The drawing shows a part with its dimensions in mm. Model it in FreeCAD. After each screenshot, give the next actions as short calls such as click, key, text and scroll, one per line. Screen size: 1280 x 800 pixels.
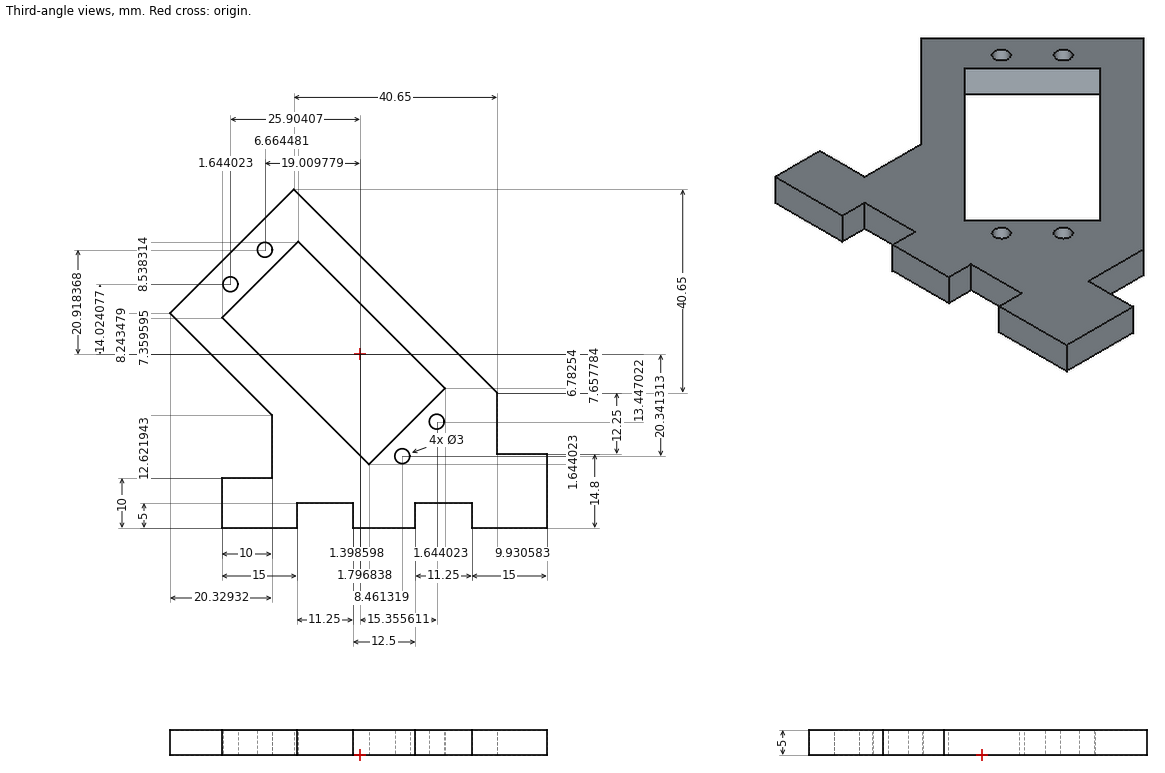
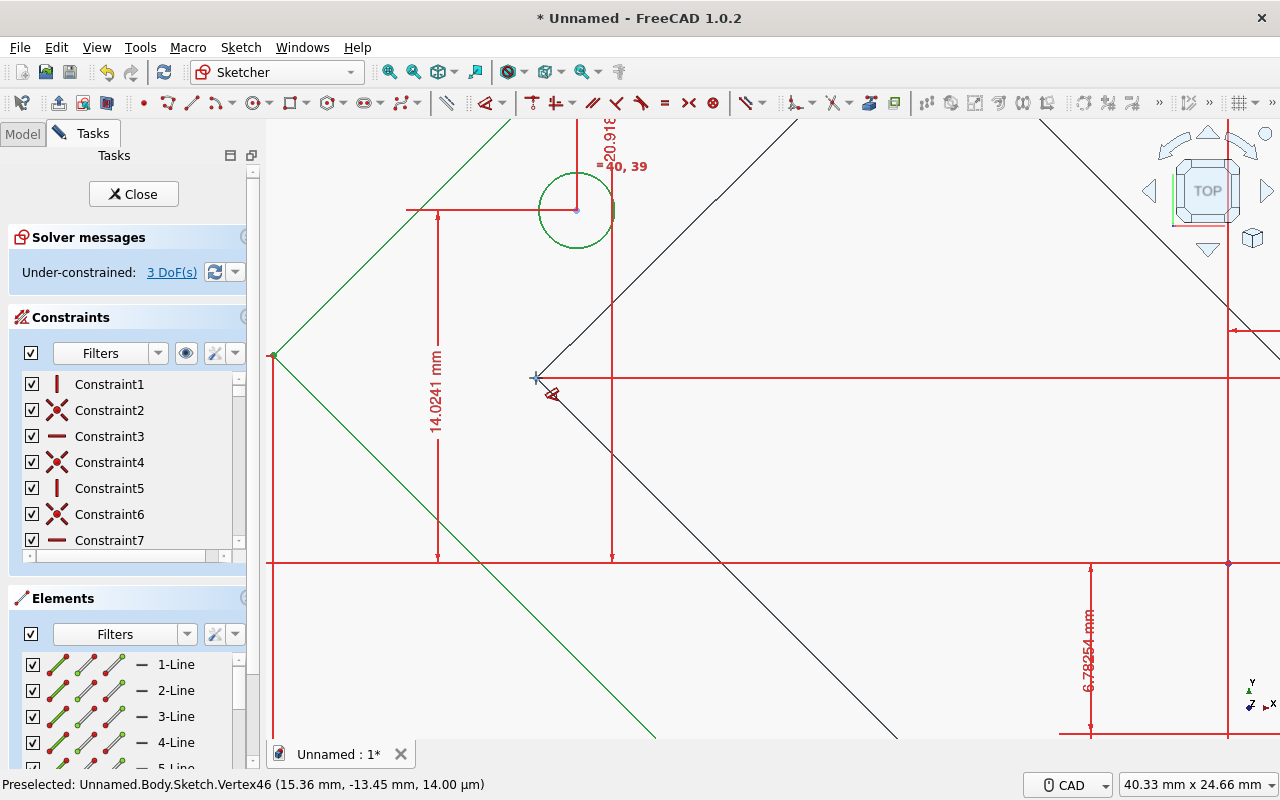
click(537, 378)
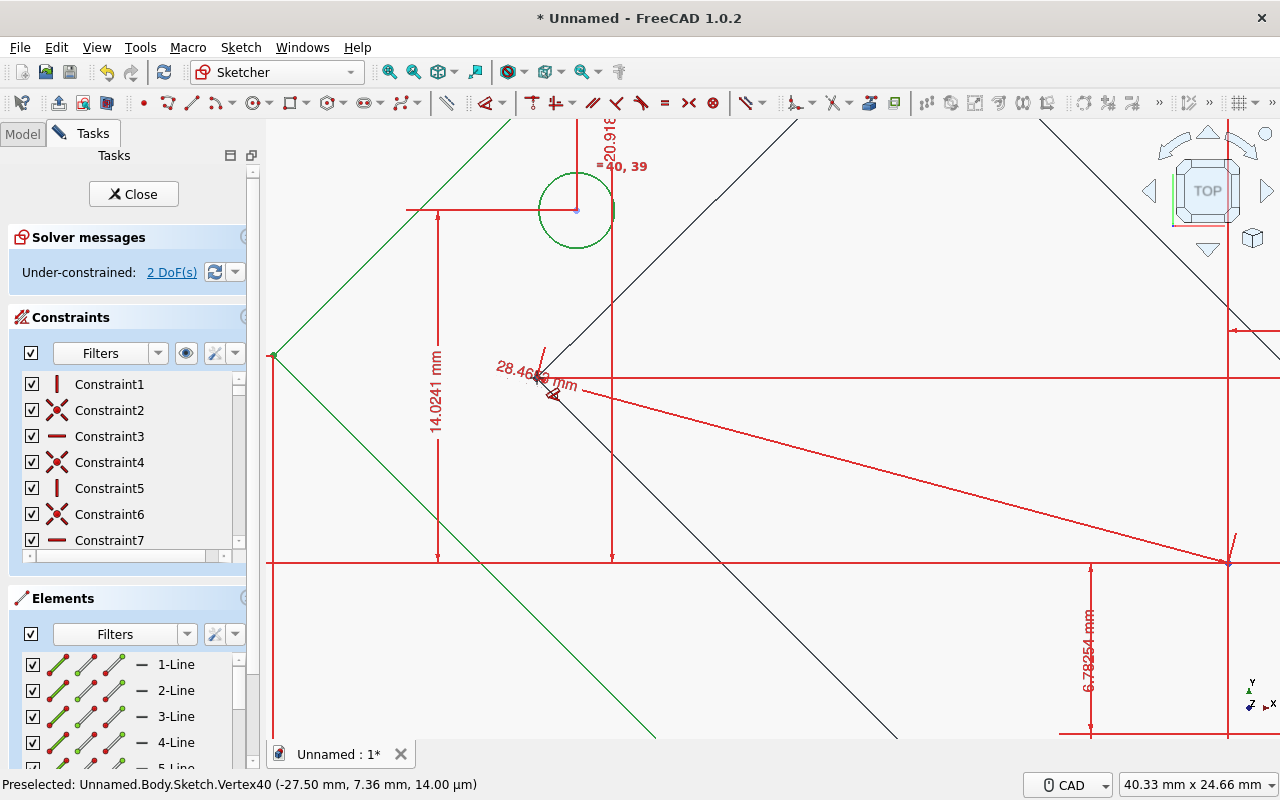
click(577, 210)
click(548, 412)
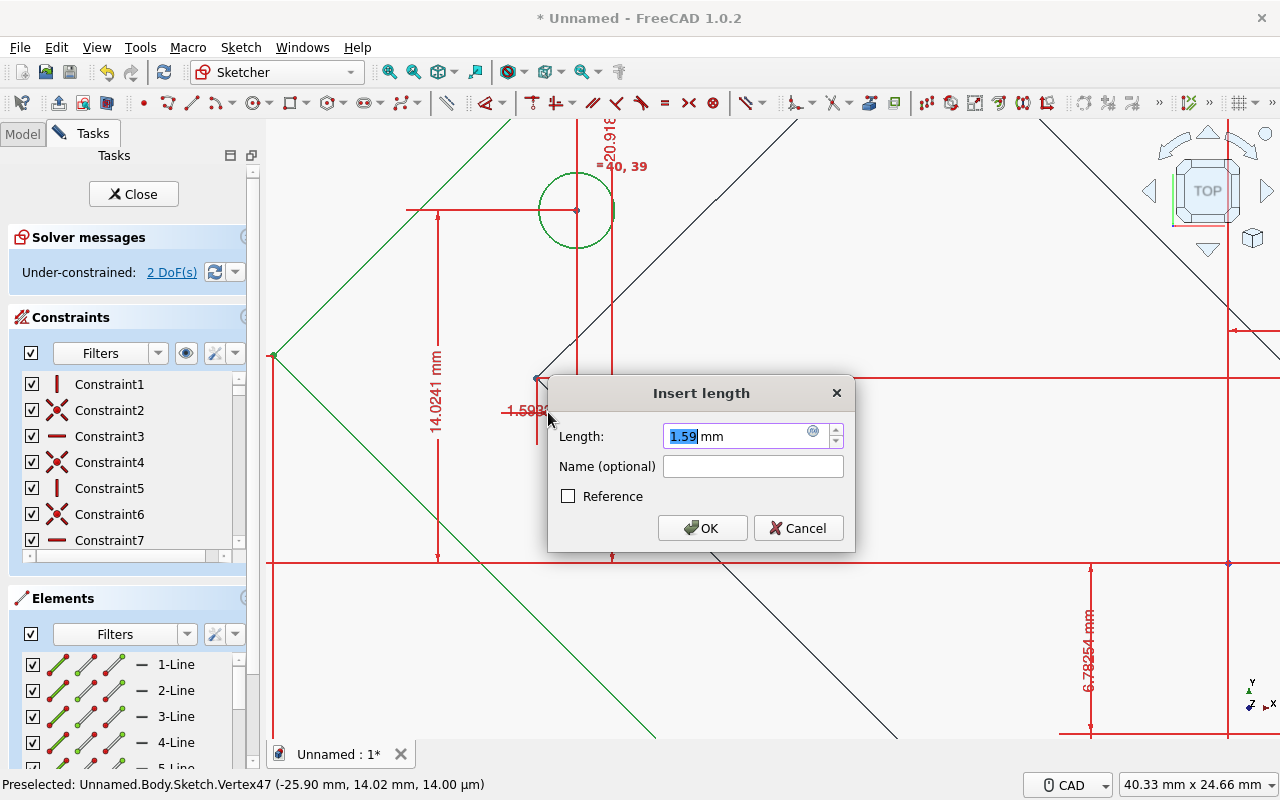
text(1.644023)
key(Return)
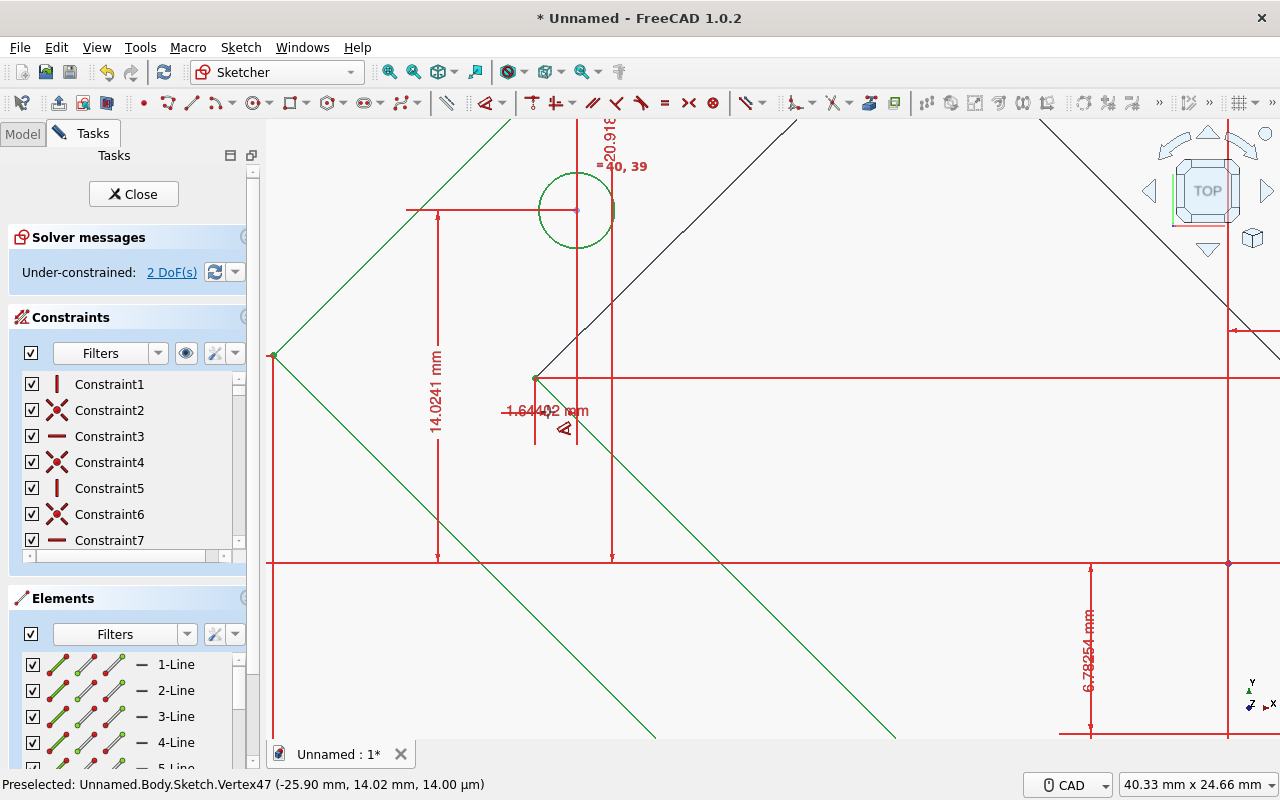
scroll(536, 378, down, 7)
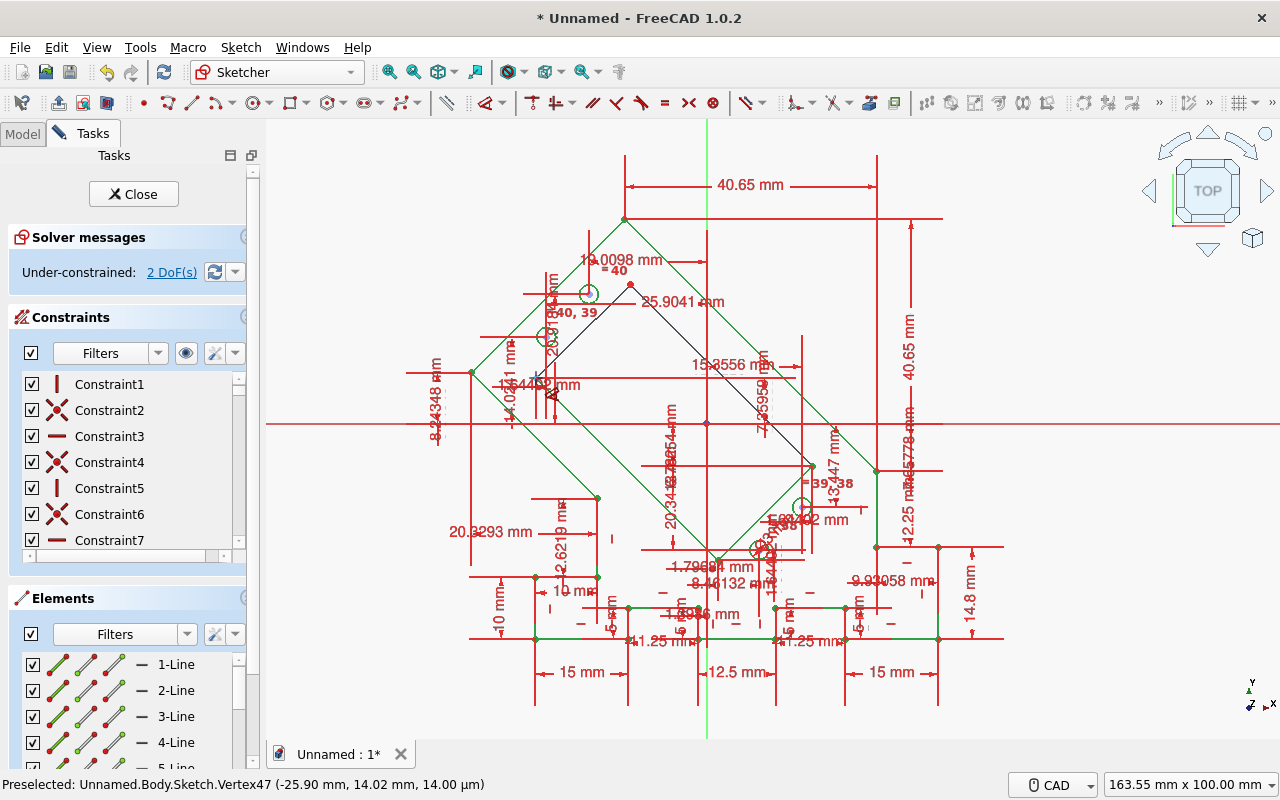
click(631, 285)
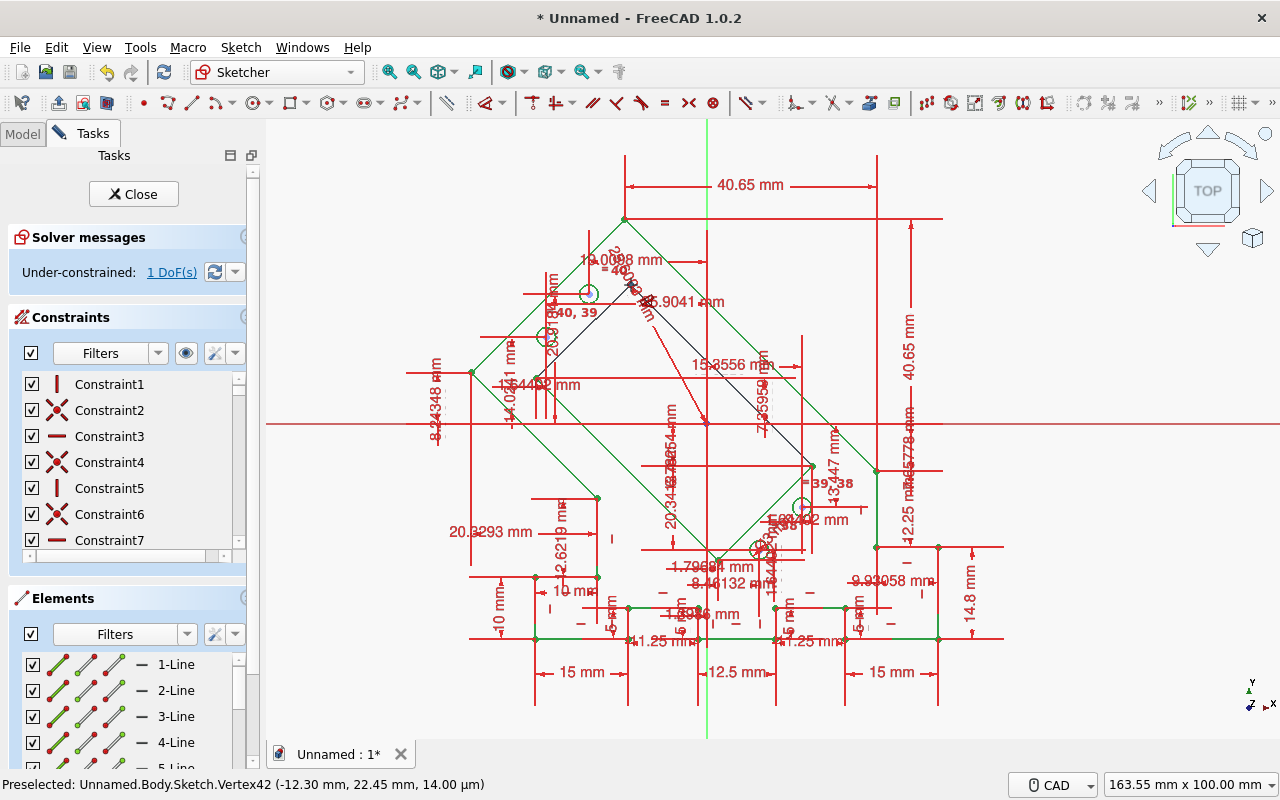
click(546, 337)
click(512, 293)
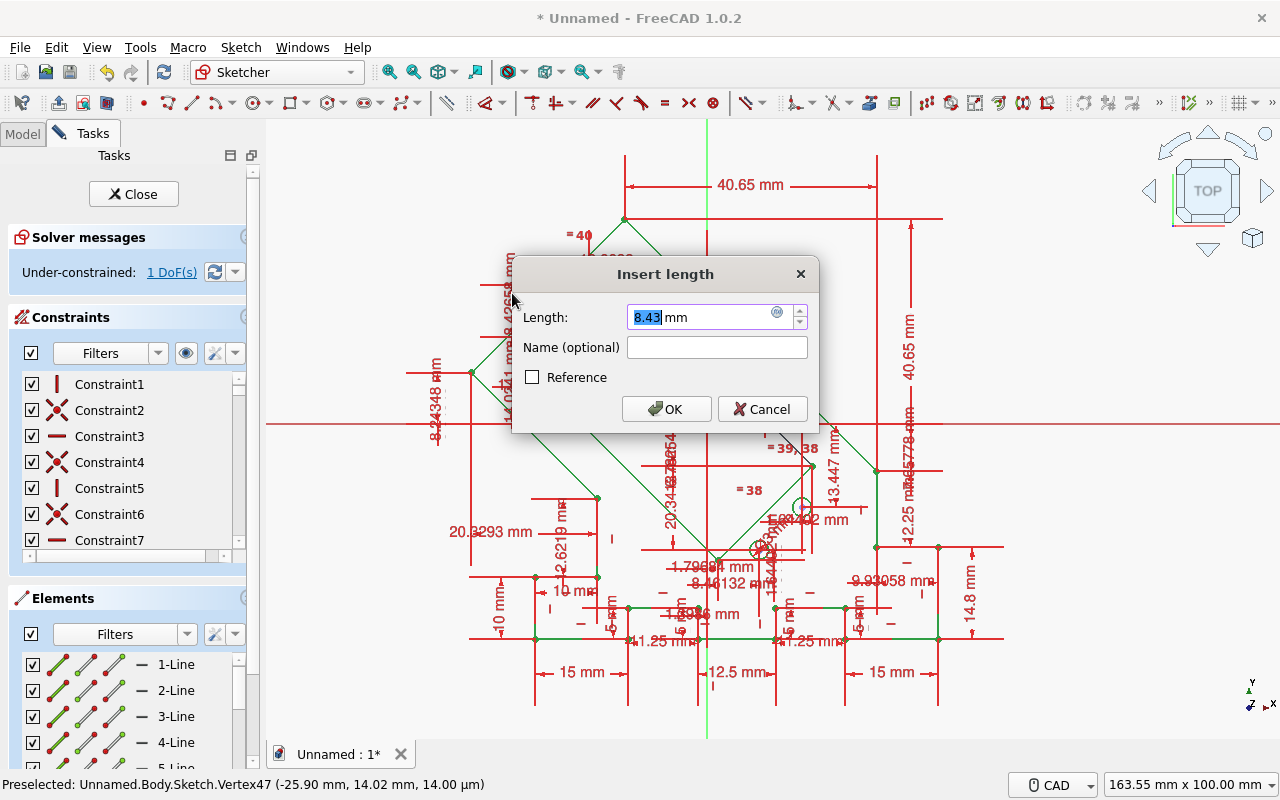
text(8.538314)
key(Return)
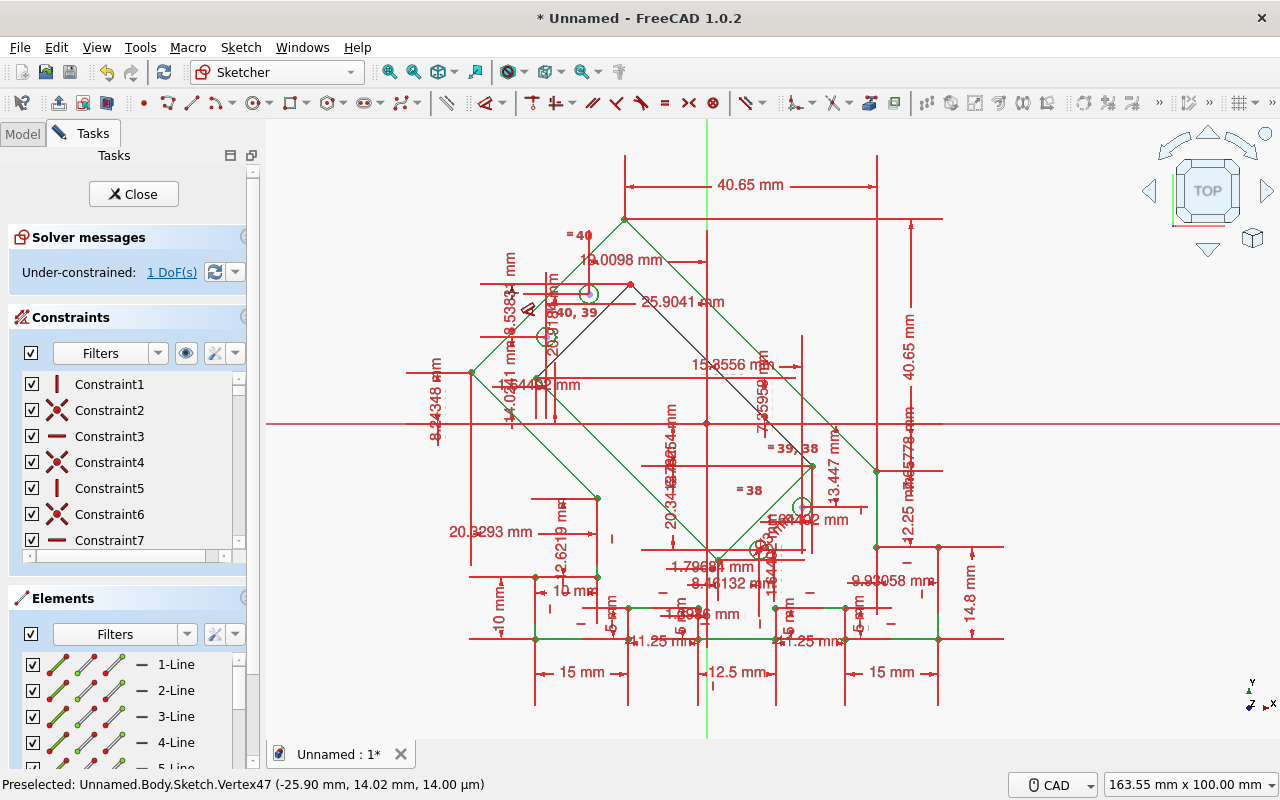
click(631, 284)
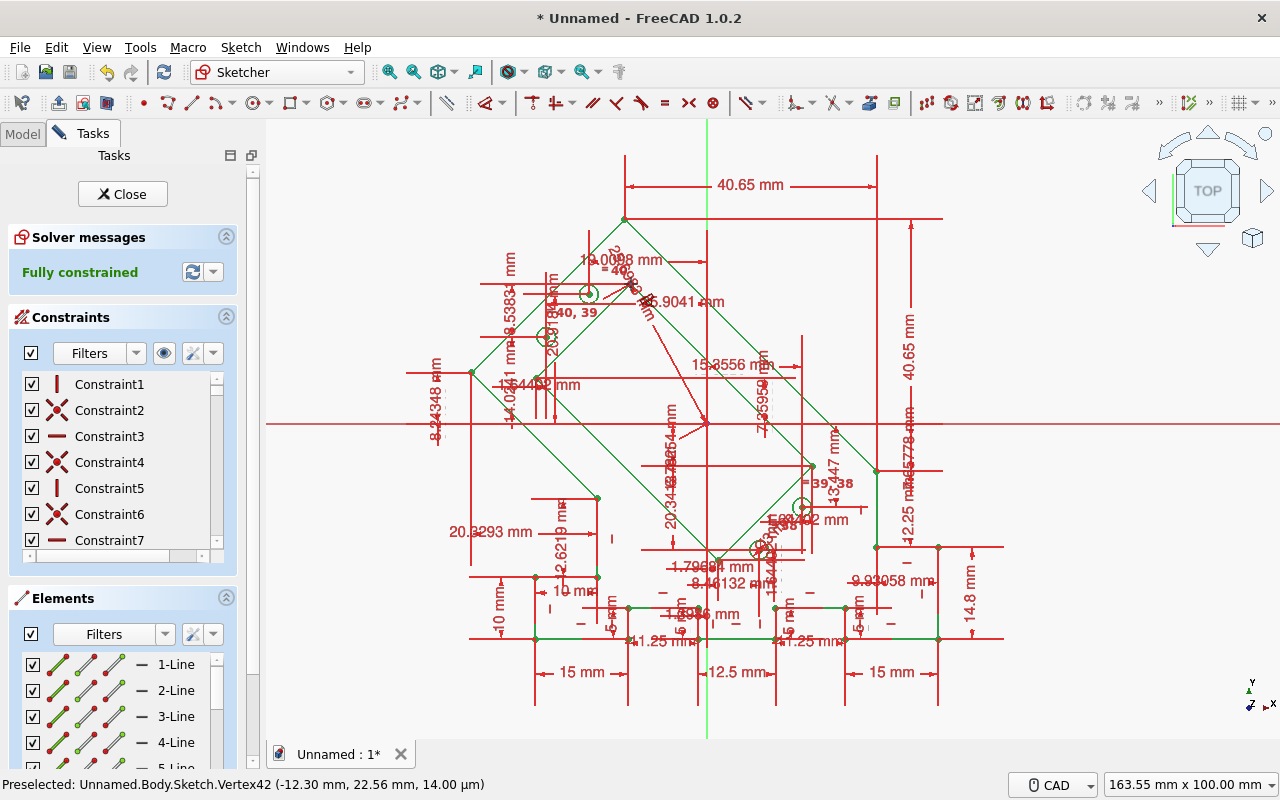
click(589, 294)
click(595, 226)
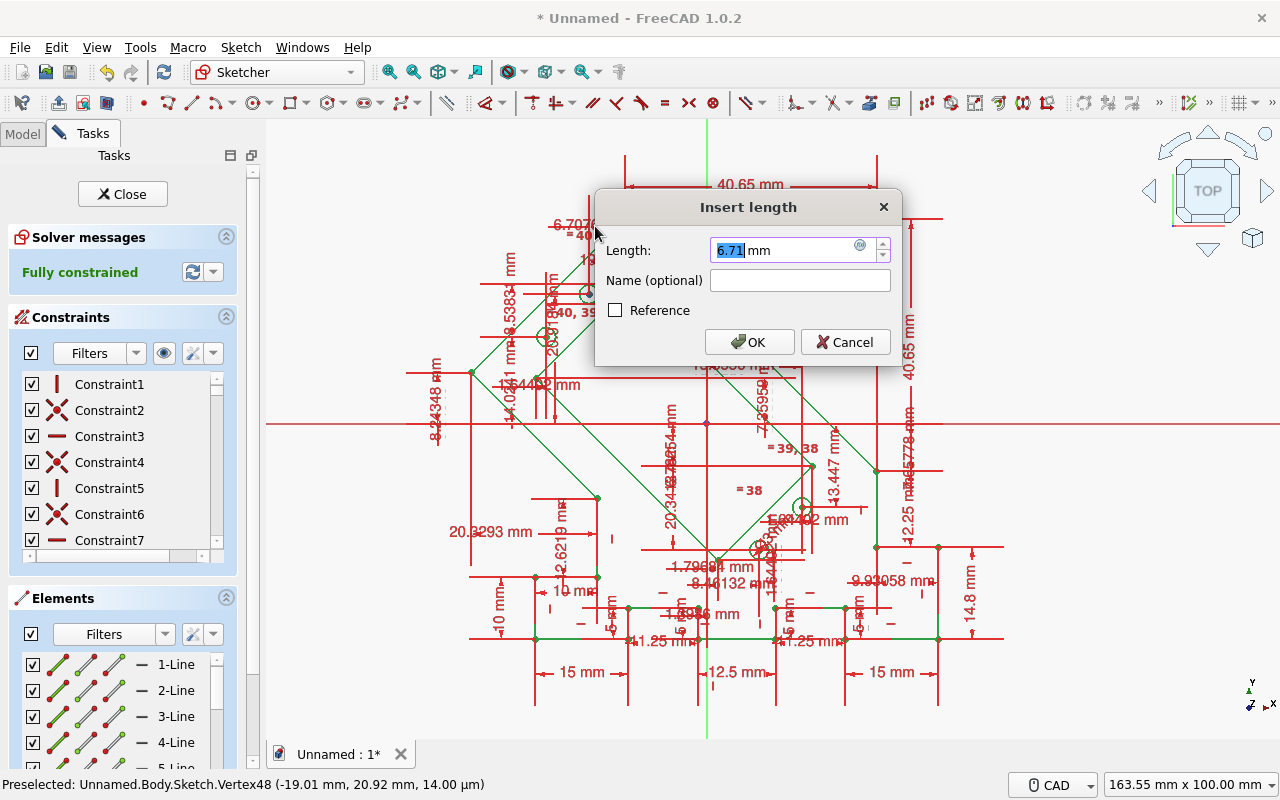
text(6.664481)
key(Return)
key(Escape)